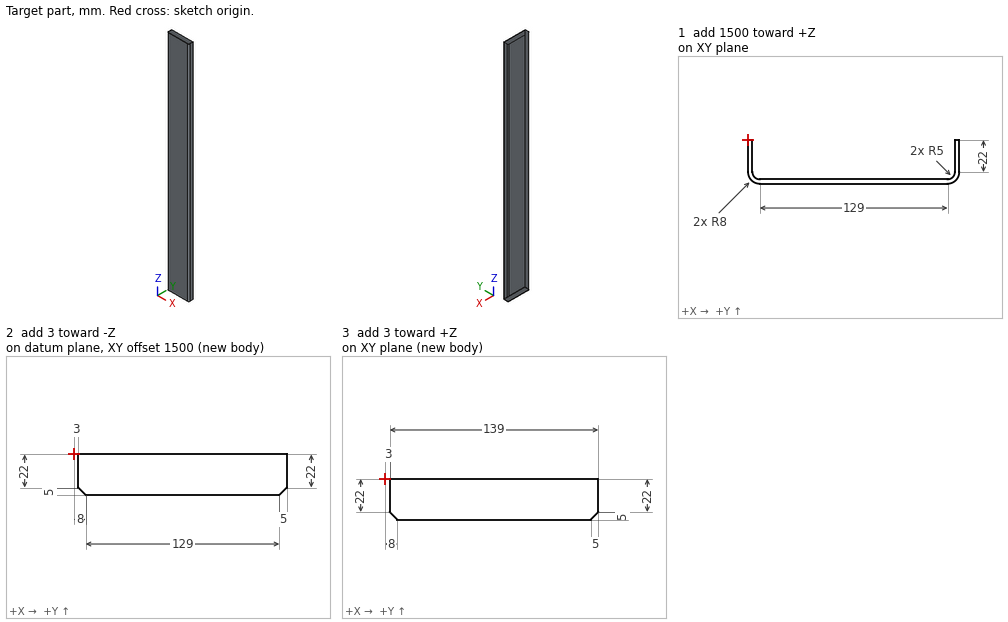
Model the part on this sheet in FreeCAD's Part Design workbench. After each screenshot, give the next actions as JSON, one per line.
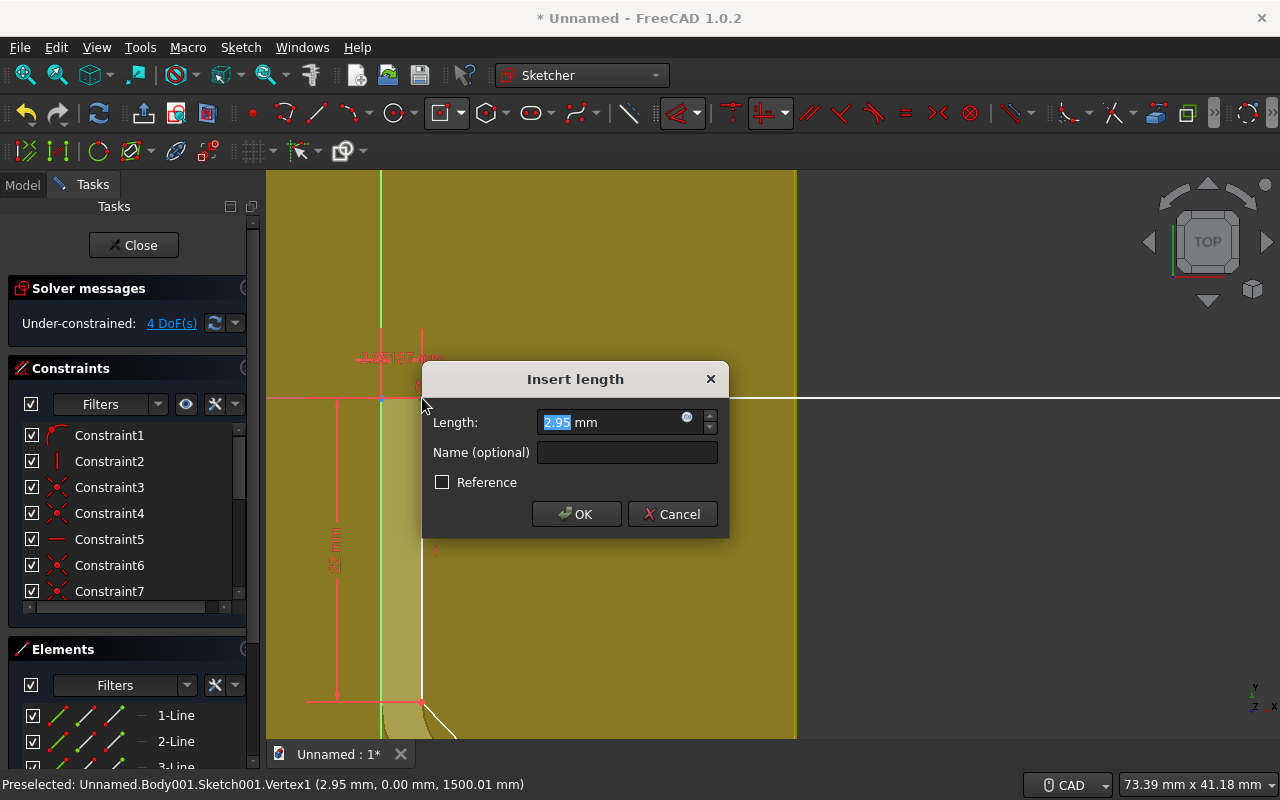
{"action": "type", "text": "3"}
{"action": "key", "text": "Return"}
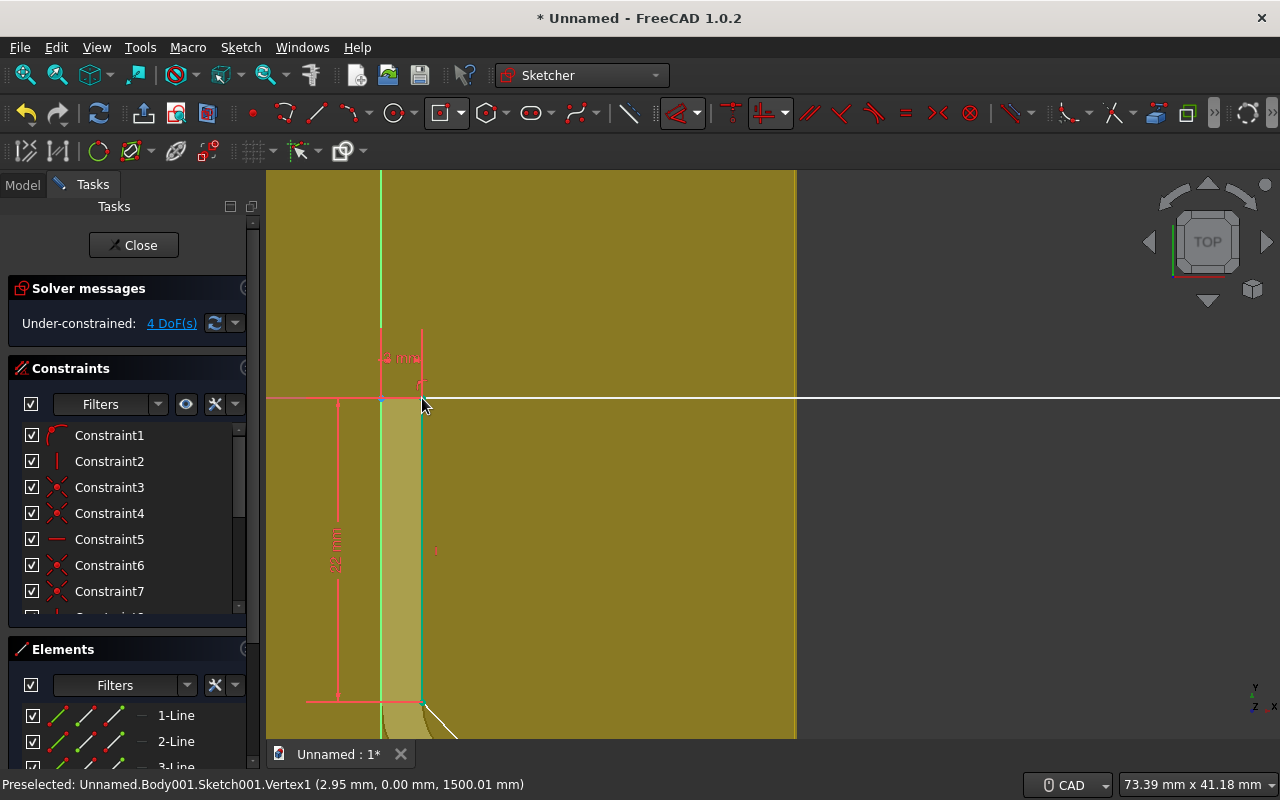
{"action": "scroll", "coordinate": [421, 398], "scroll_direction": "down", "scroll_amount": 6}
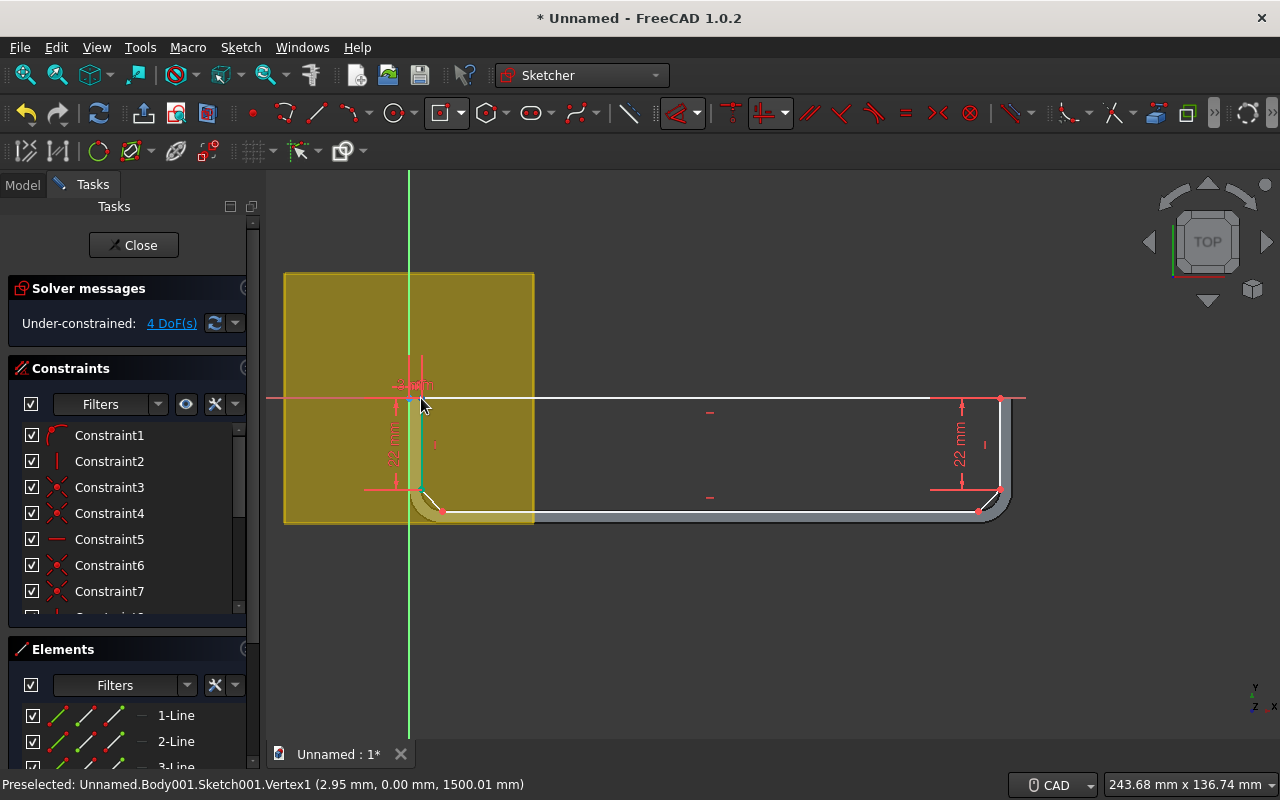
{"action": "left_click", "coordinate": [442, 512]}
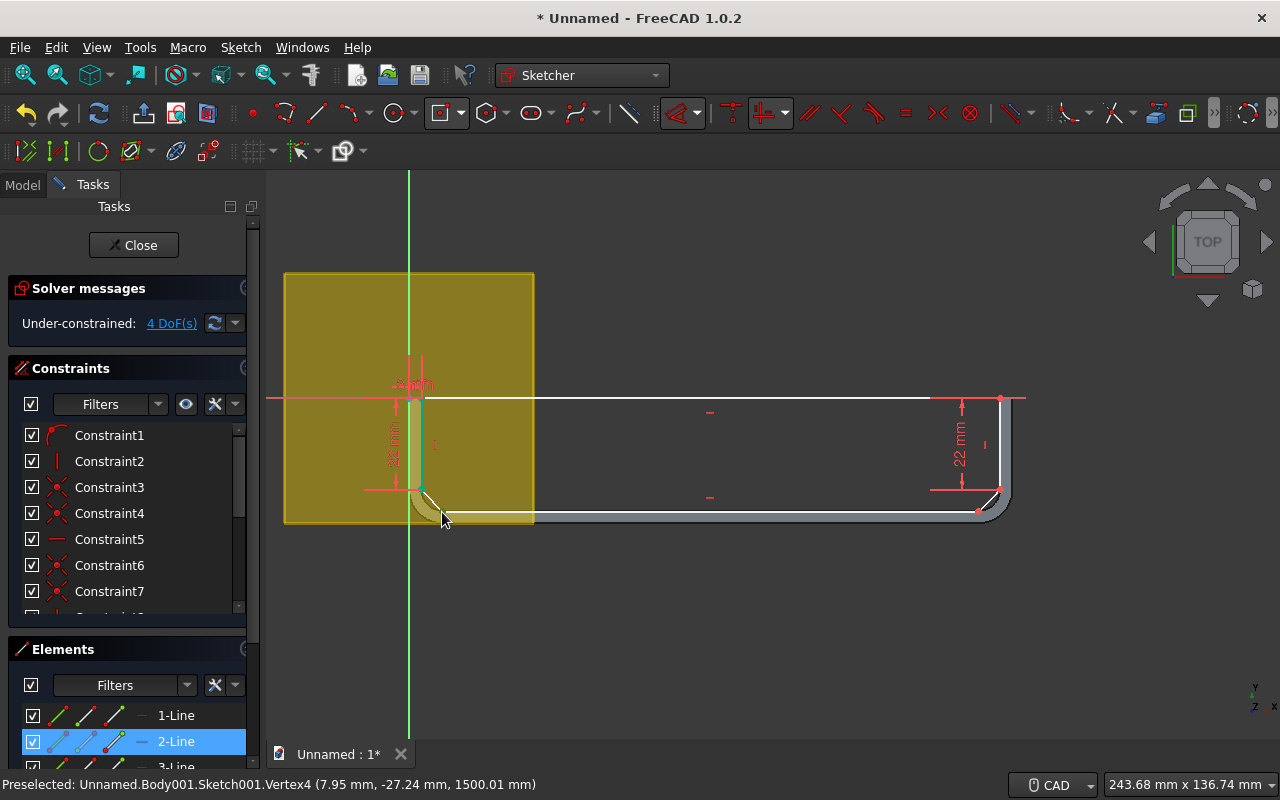
{"action": "key", "text": "l"}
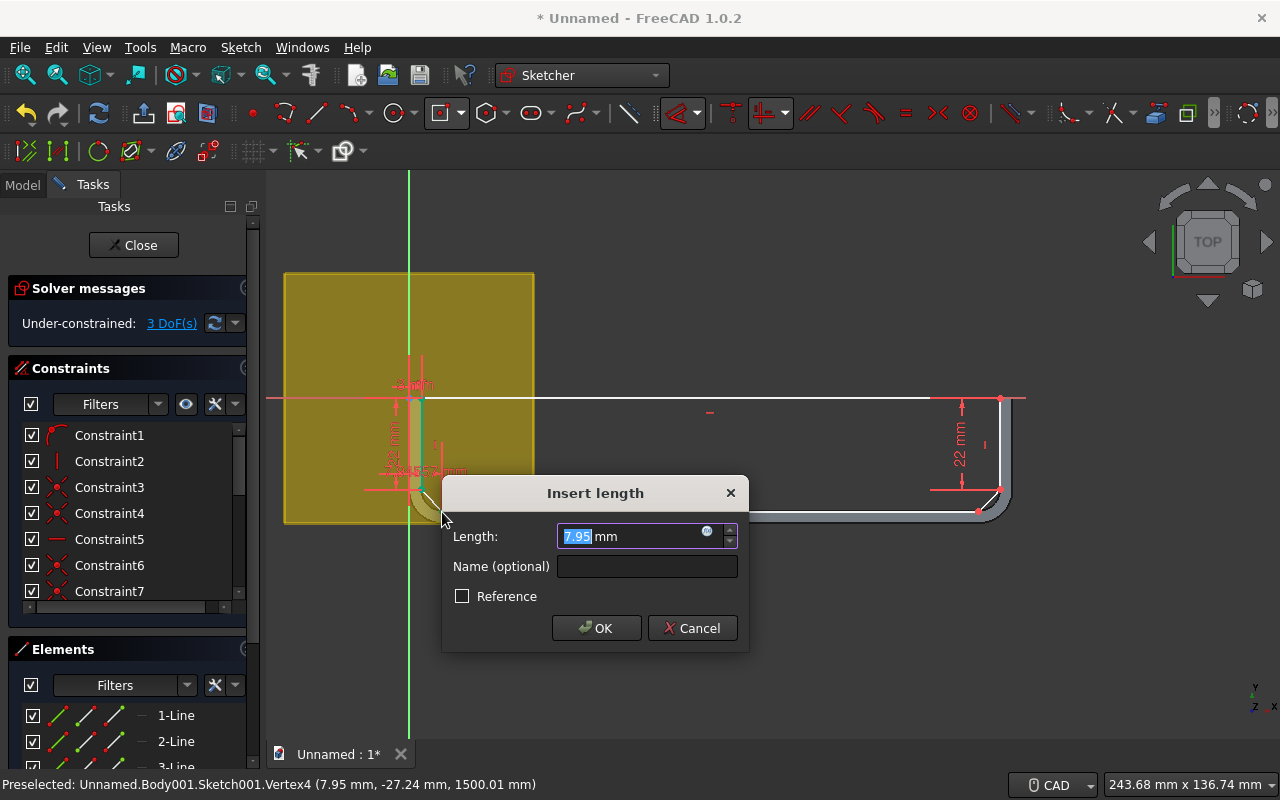
{"action": "type", "text": "8"}
{"action": "key", "text": "Return"}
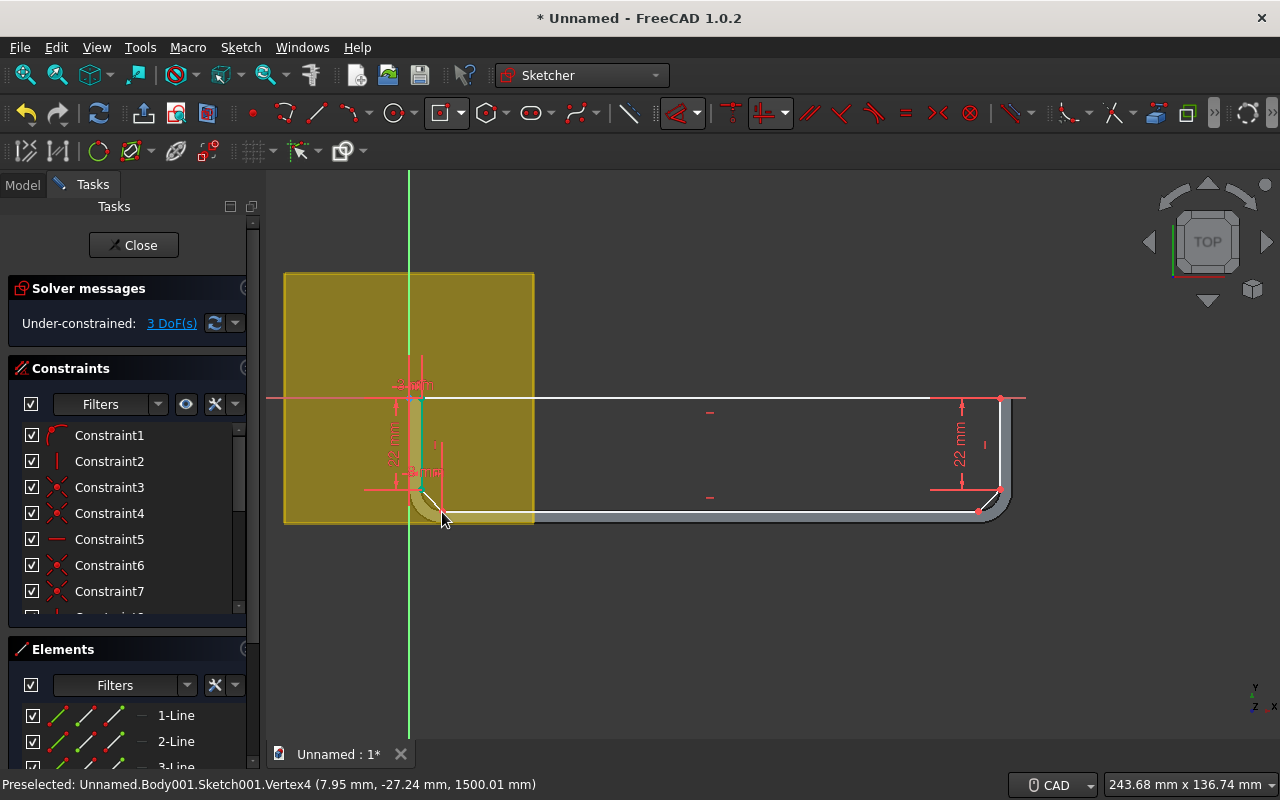
{"action": "scroll", "coordinate": [428, 496], "scroll_direction": "up", "scroll_amount": 4}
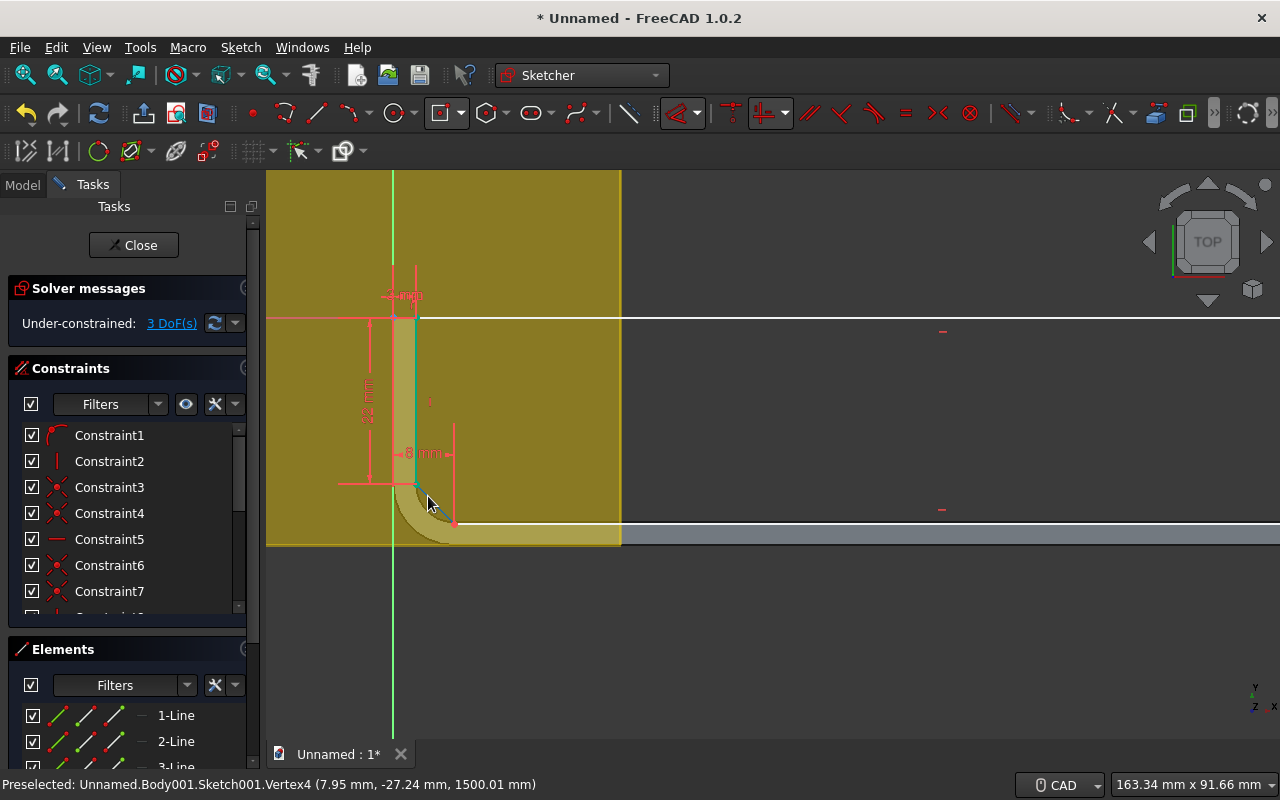
{"action": "left_click", "coordinate": [427, 496]}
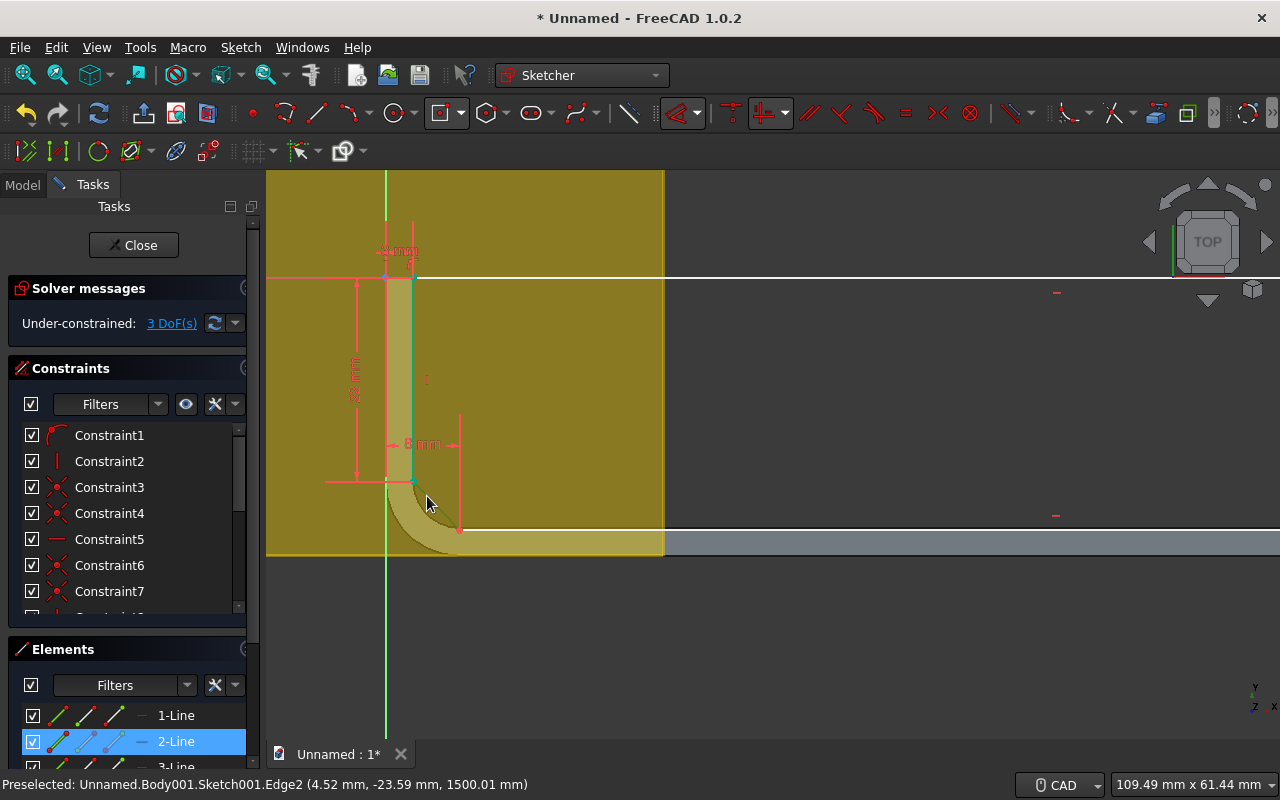
{"action": "key", "text": "i"}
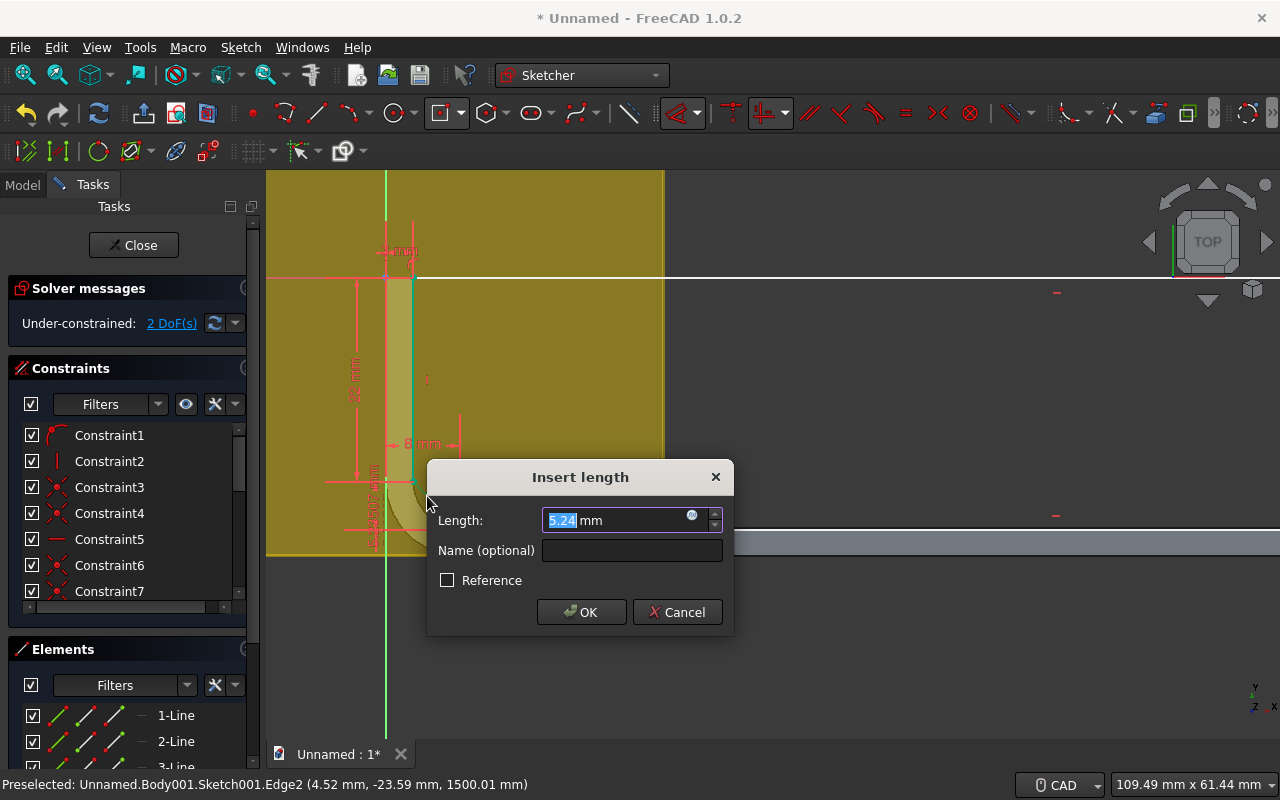
{"action": "type", "text": "5"}
{"action": "key", "text": "Return"}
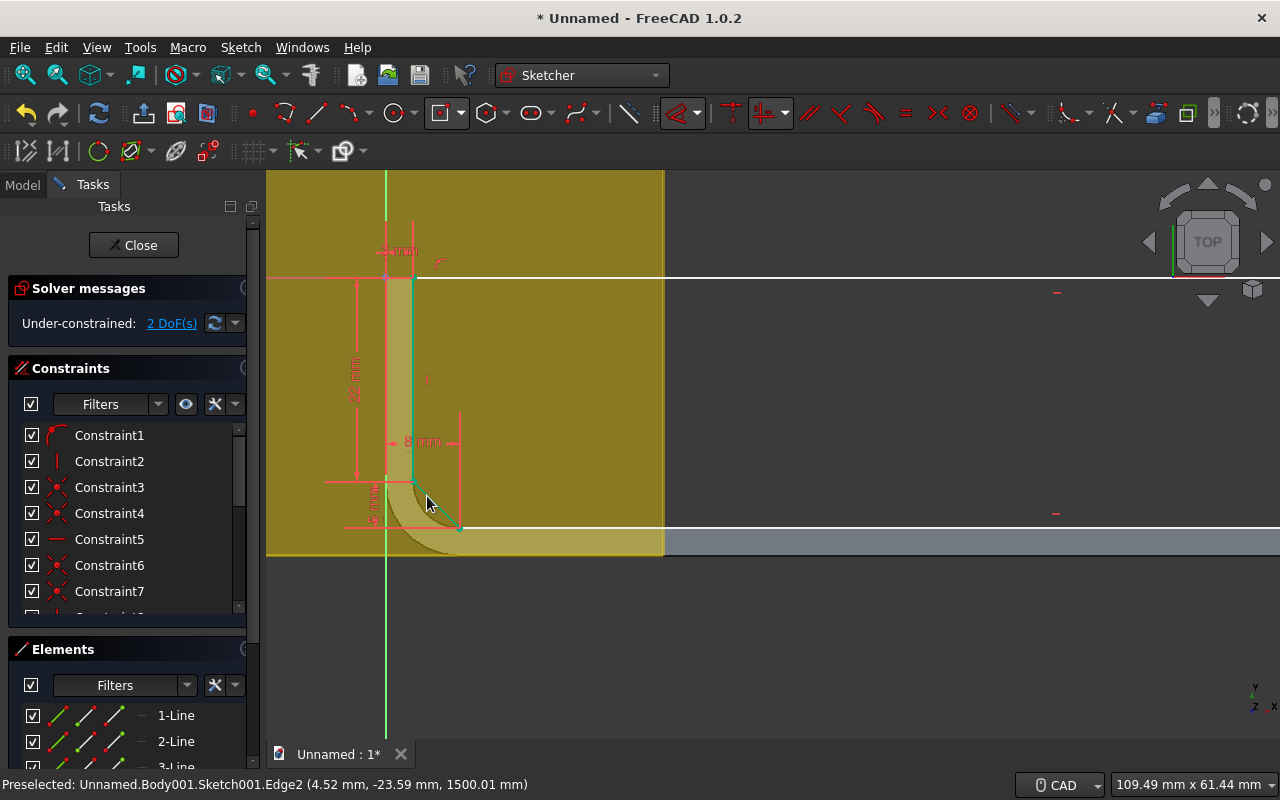
{"action": "scroll", "coordinate": [428, 497], "scroll_direction": "down", "scroll_amount": 4}